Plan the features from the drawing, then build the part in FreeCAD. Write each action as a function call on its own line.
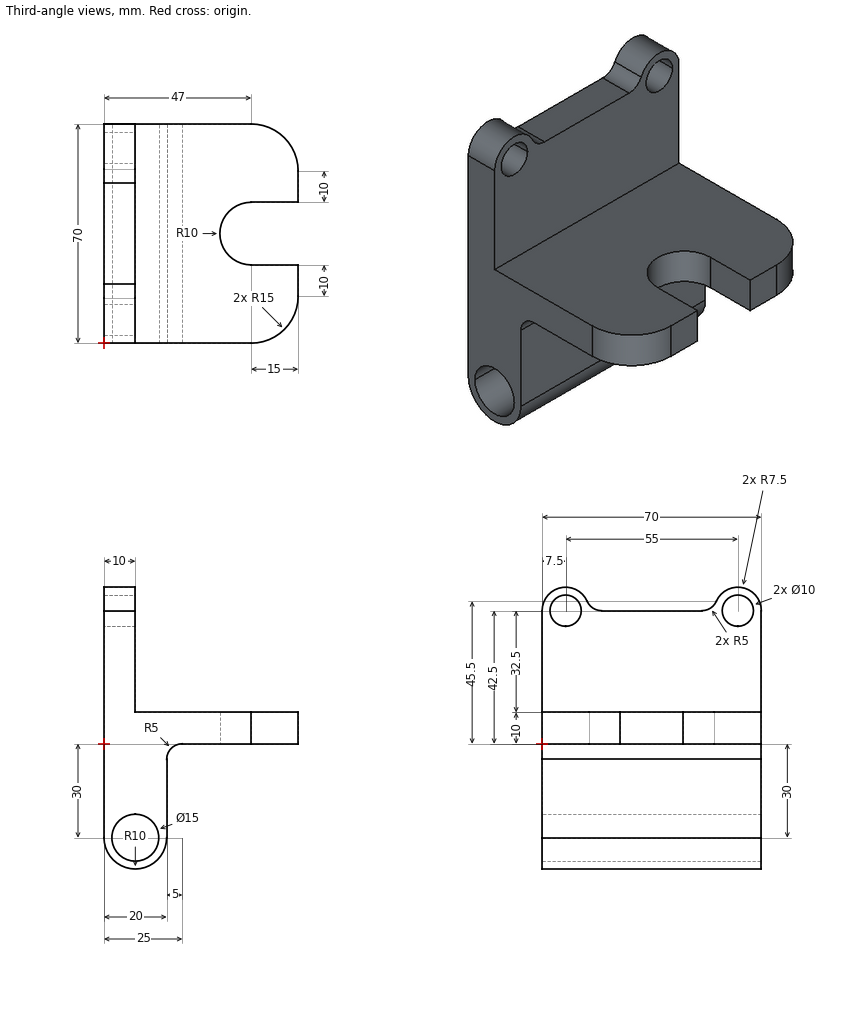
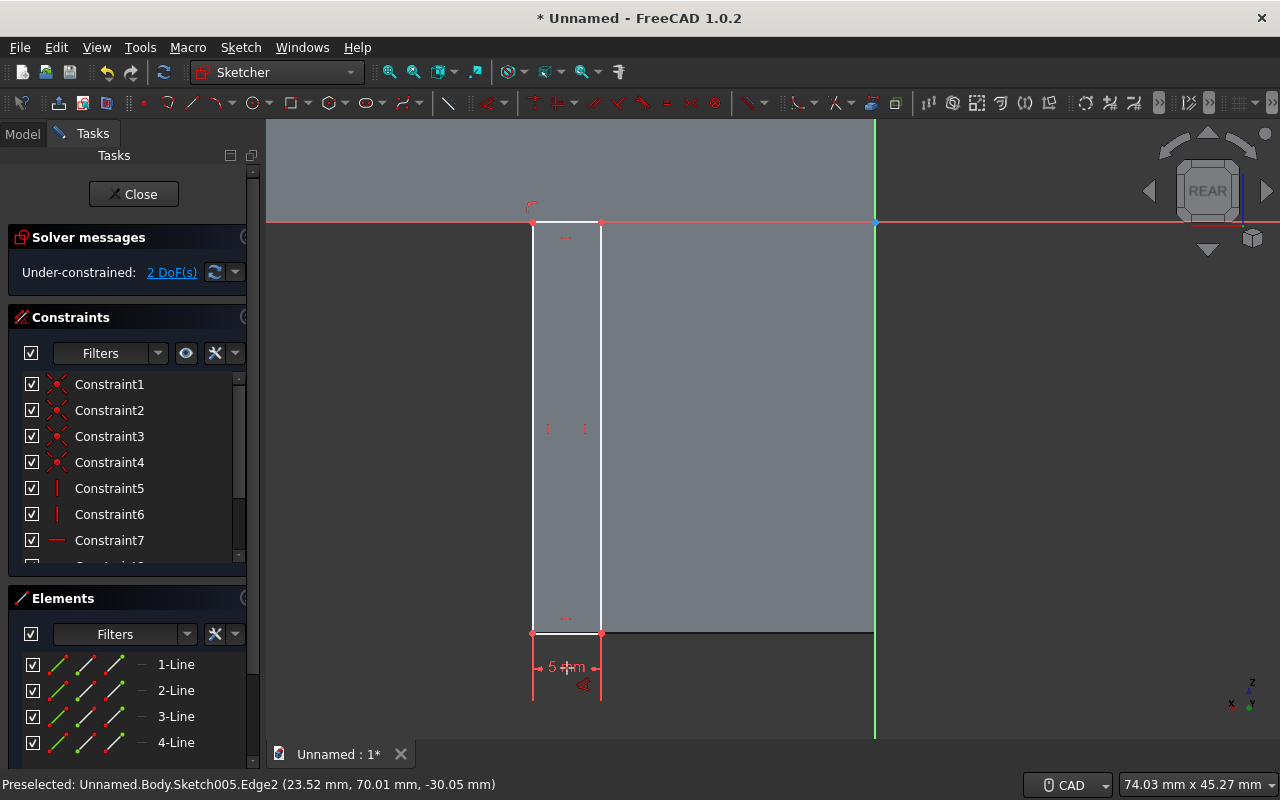
click(533, 346)
click(499, 428)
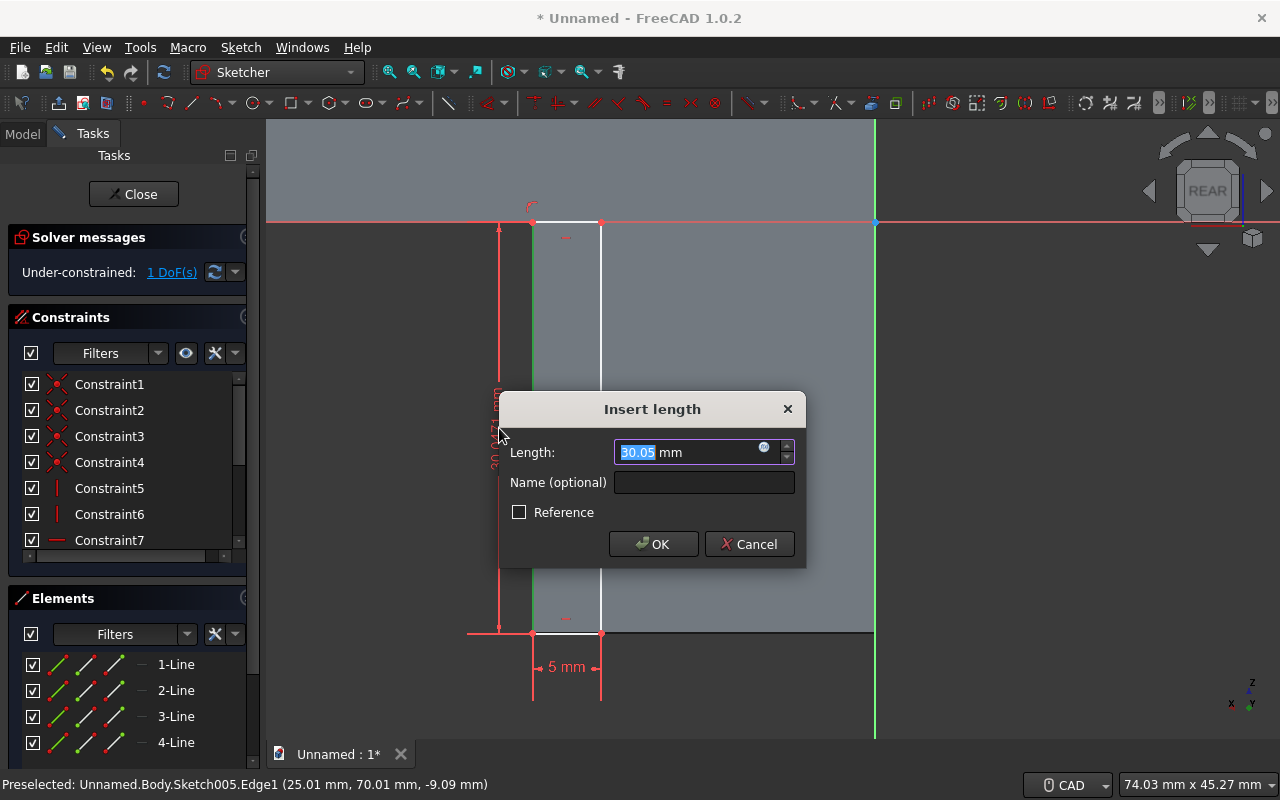
text(30)
key(Return)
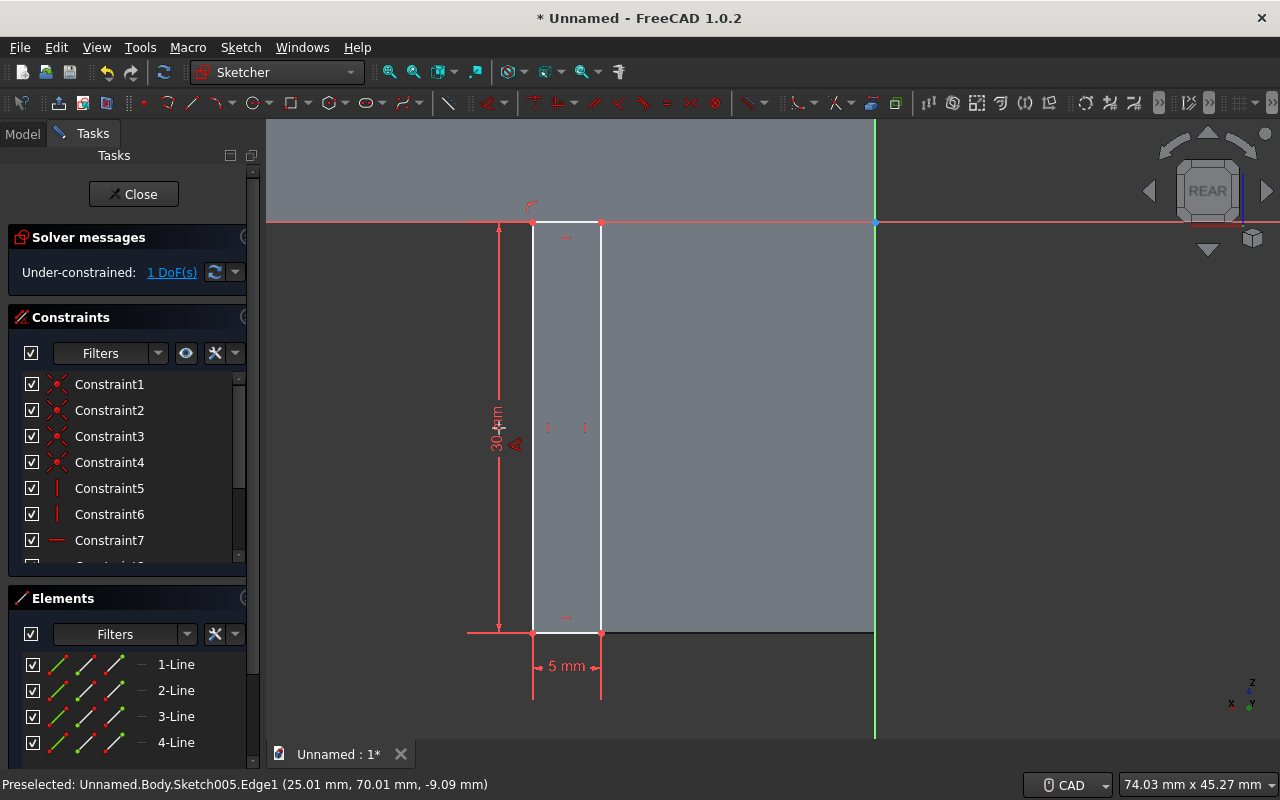
click(533, 222)
click(704, 188)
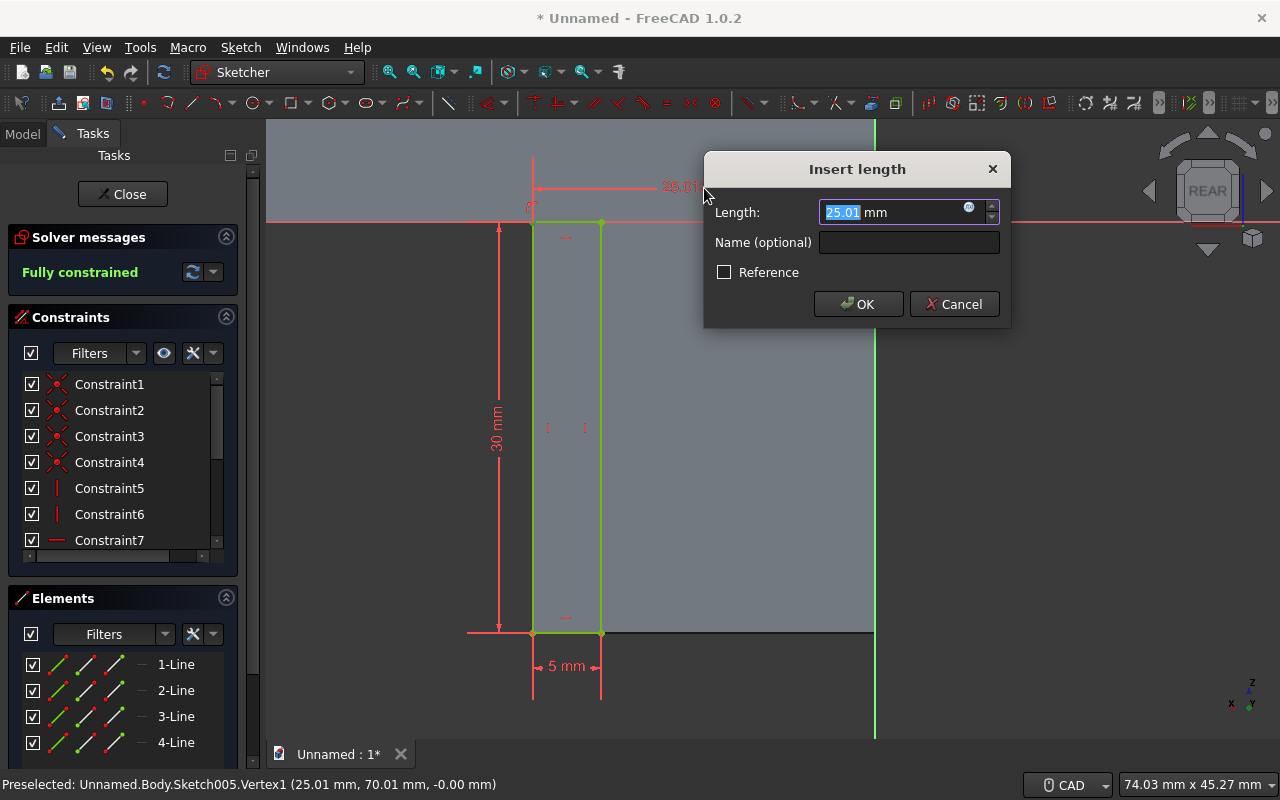
text(25)
key(Return)
key(Escape)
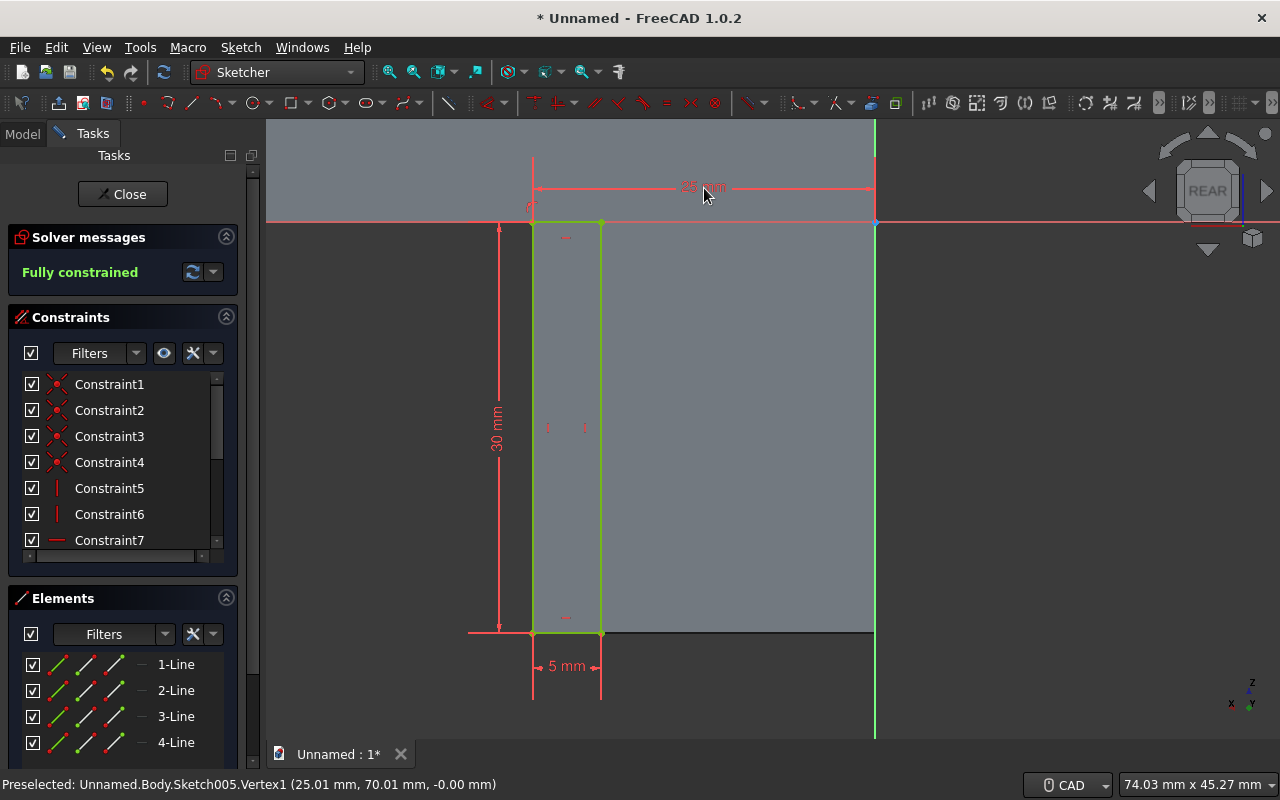
click(123, 194)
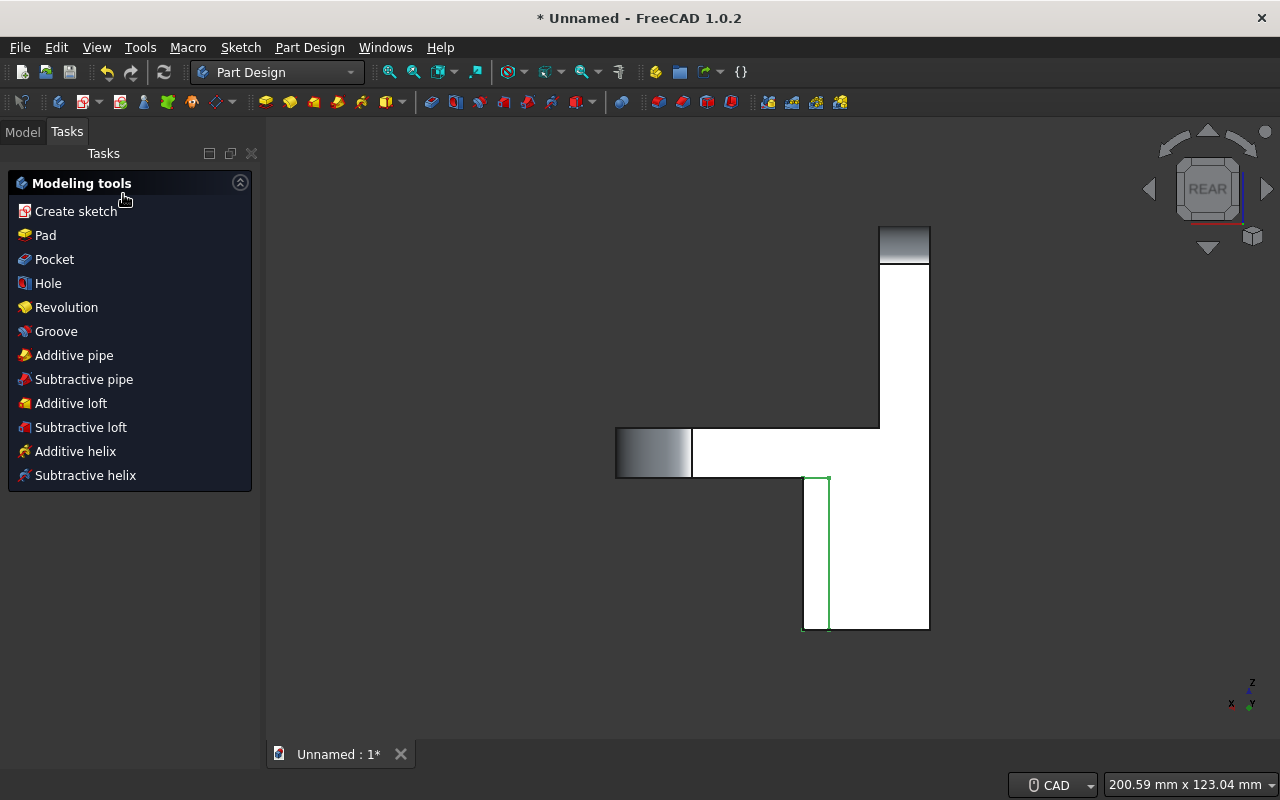
click(432, 102)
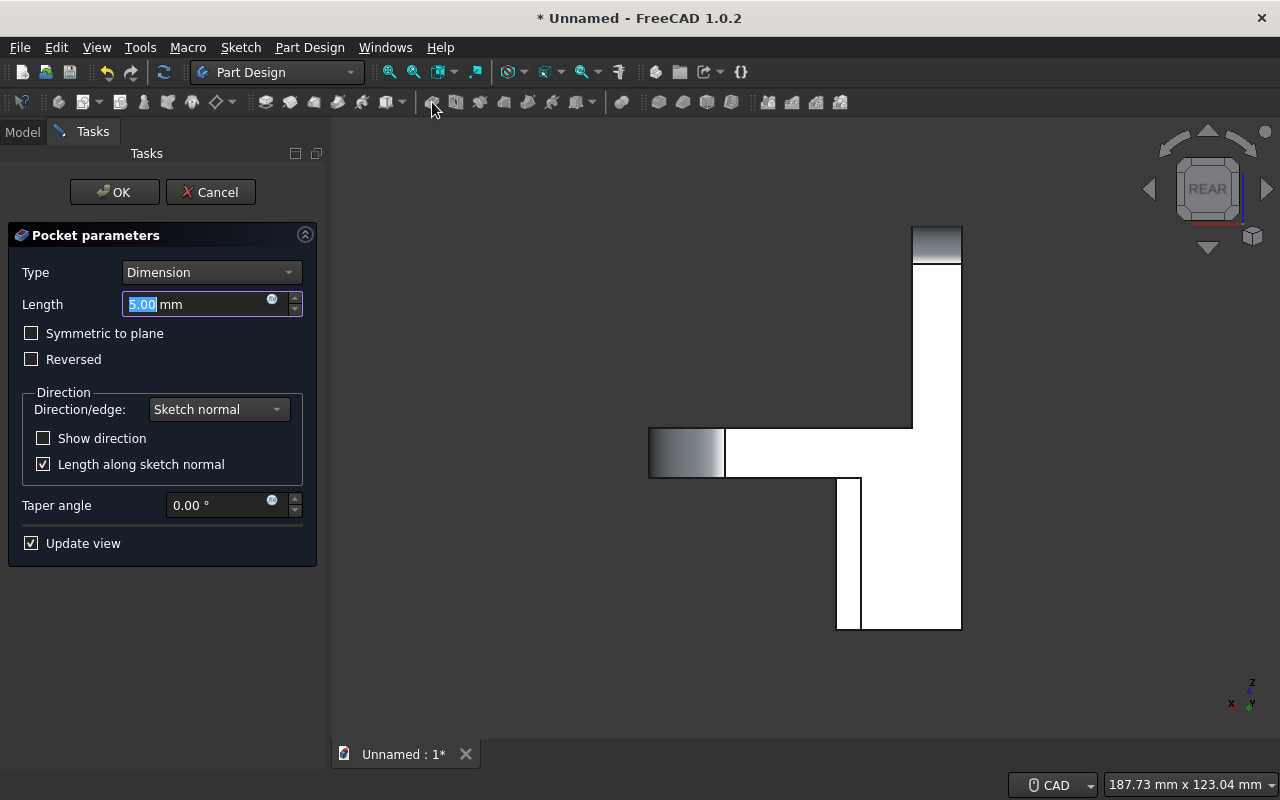
text(70)
key(Tab)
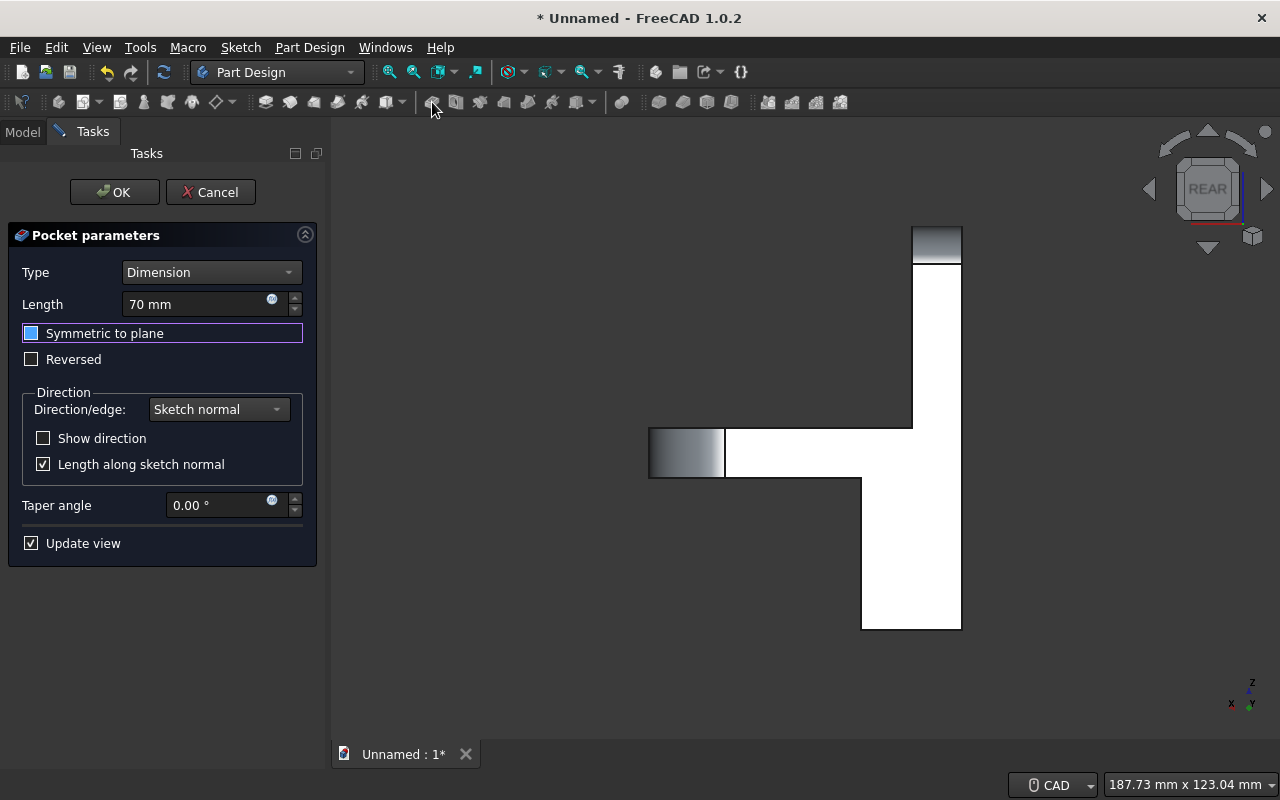
click(115, 192)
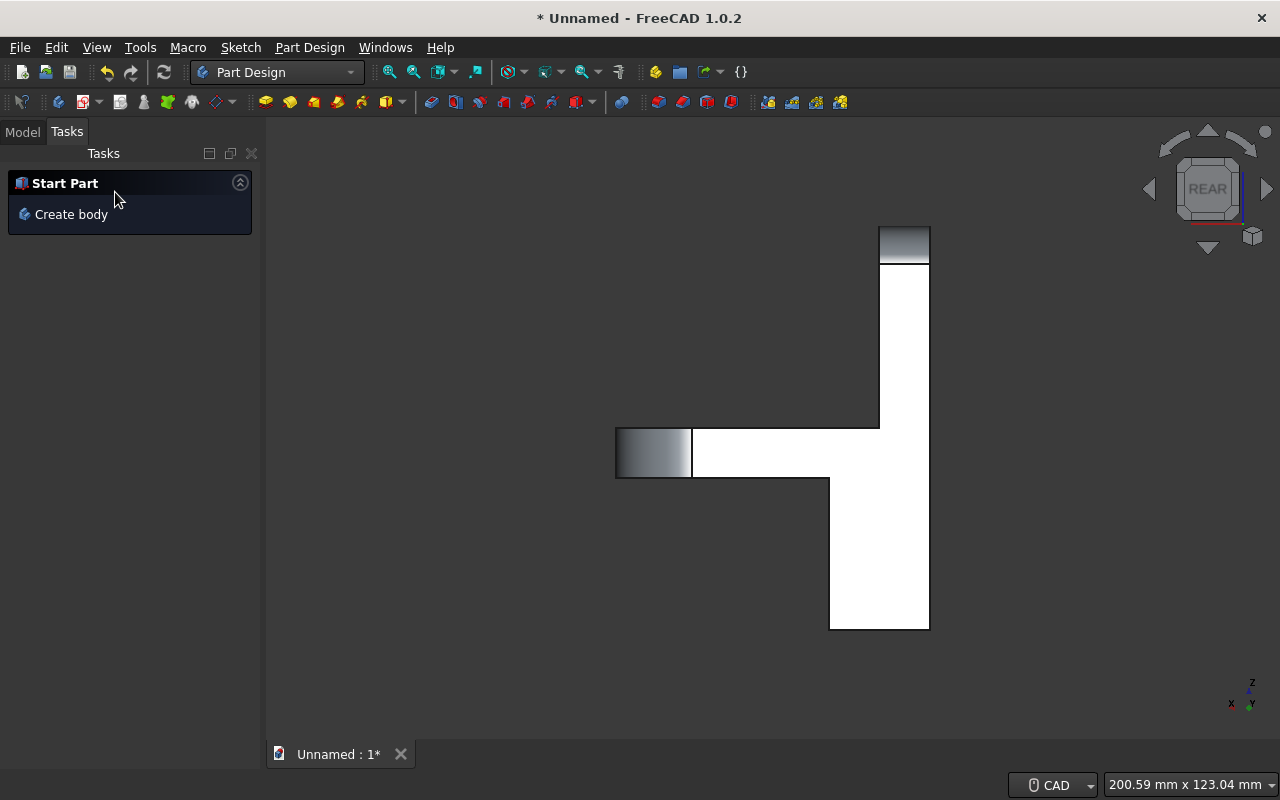
click(879, 498)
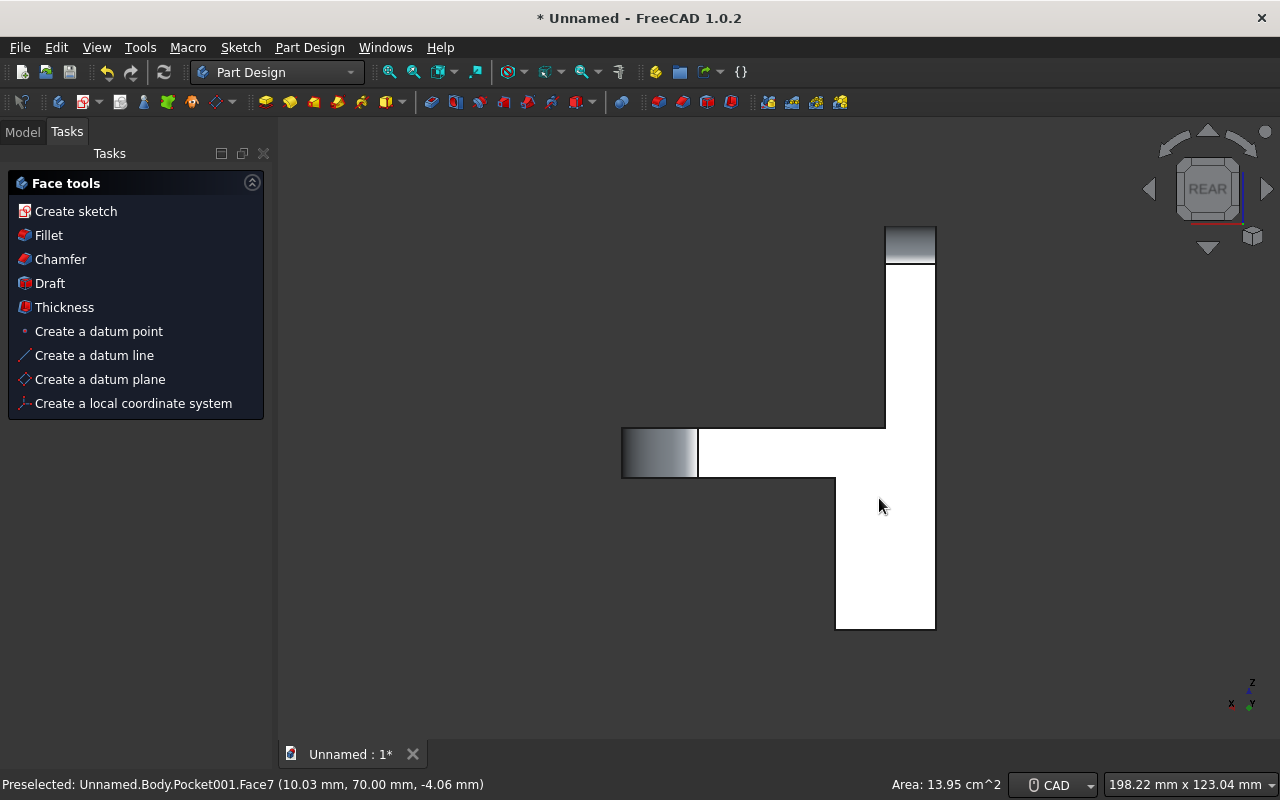
click(84, 102)